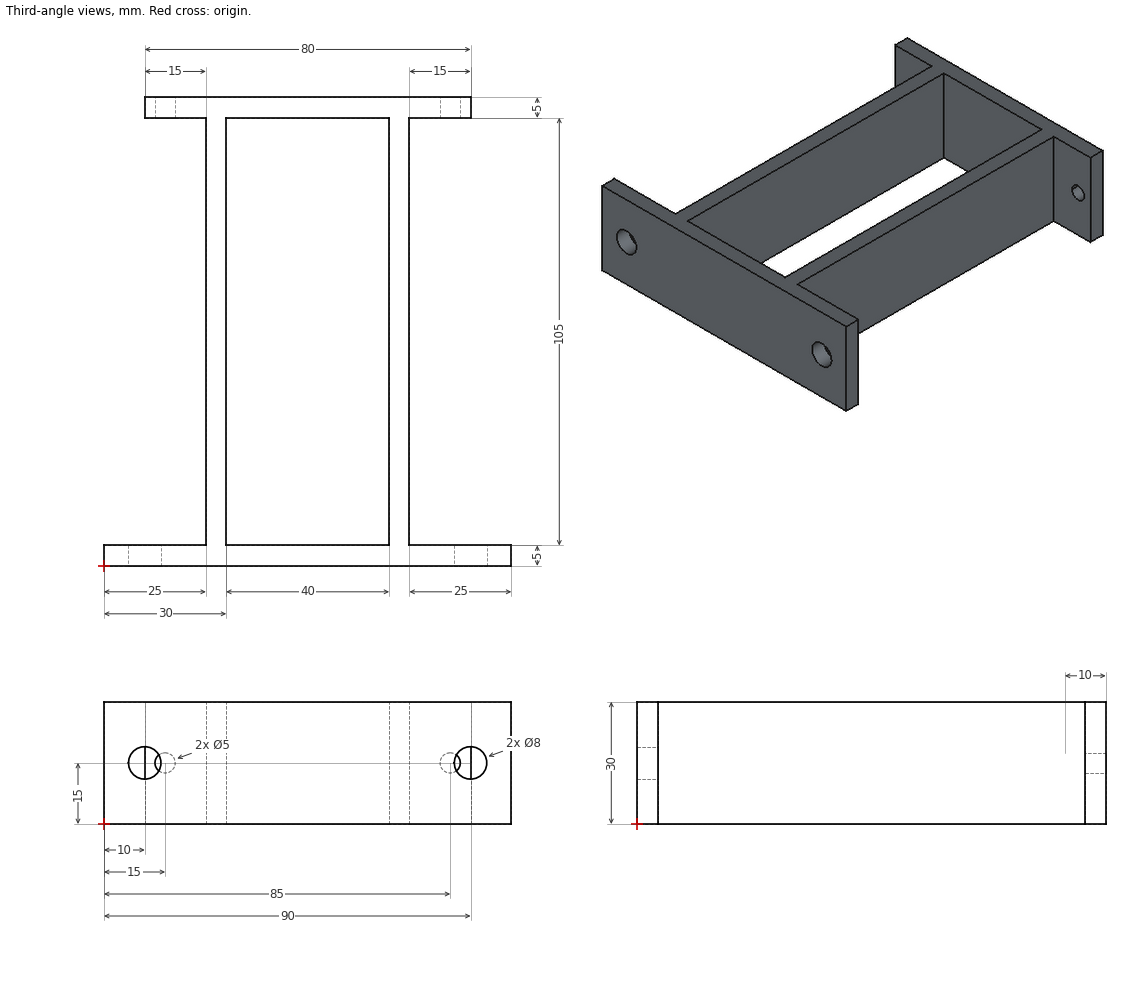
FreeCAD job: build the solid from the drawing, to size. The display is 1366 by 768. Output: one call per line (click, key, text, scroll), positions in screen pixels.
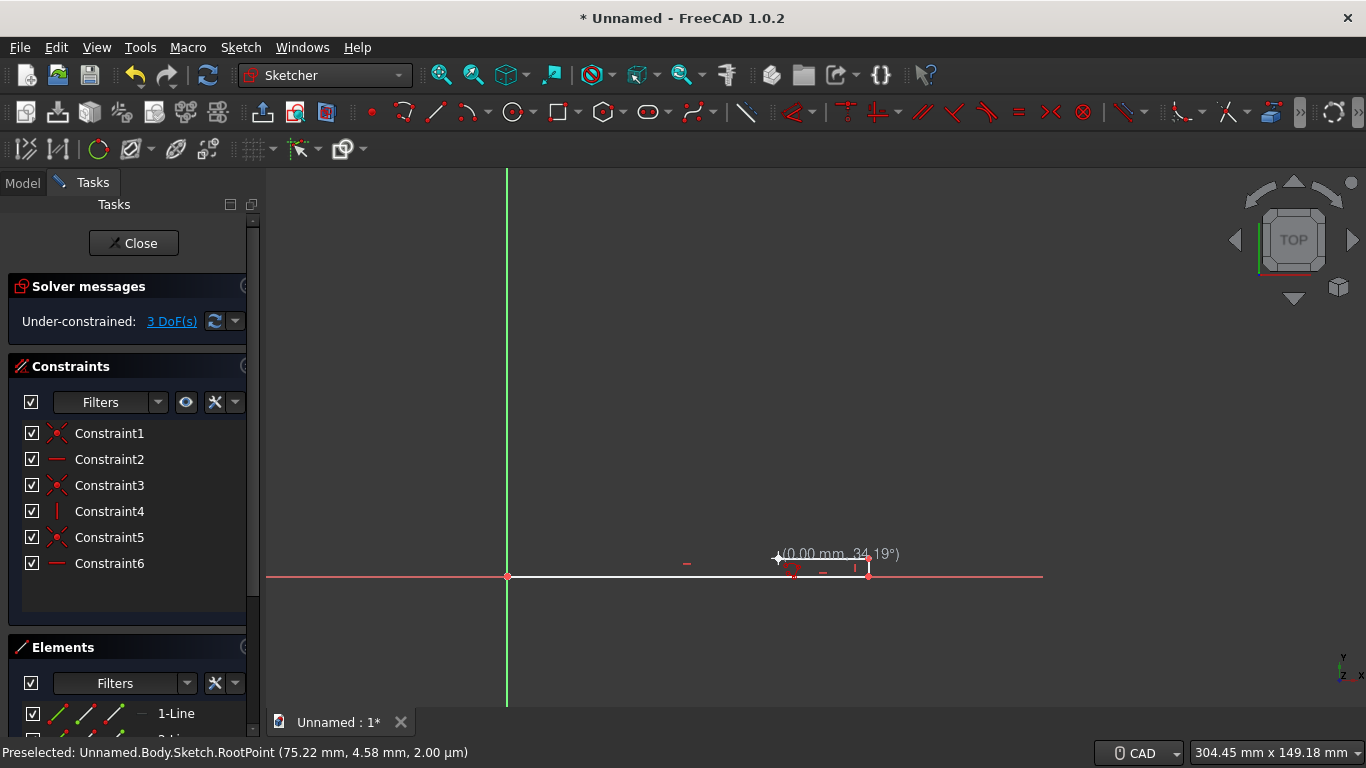
scroll(1017, 679, down, 1)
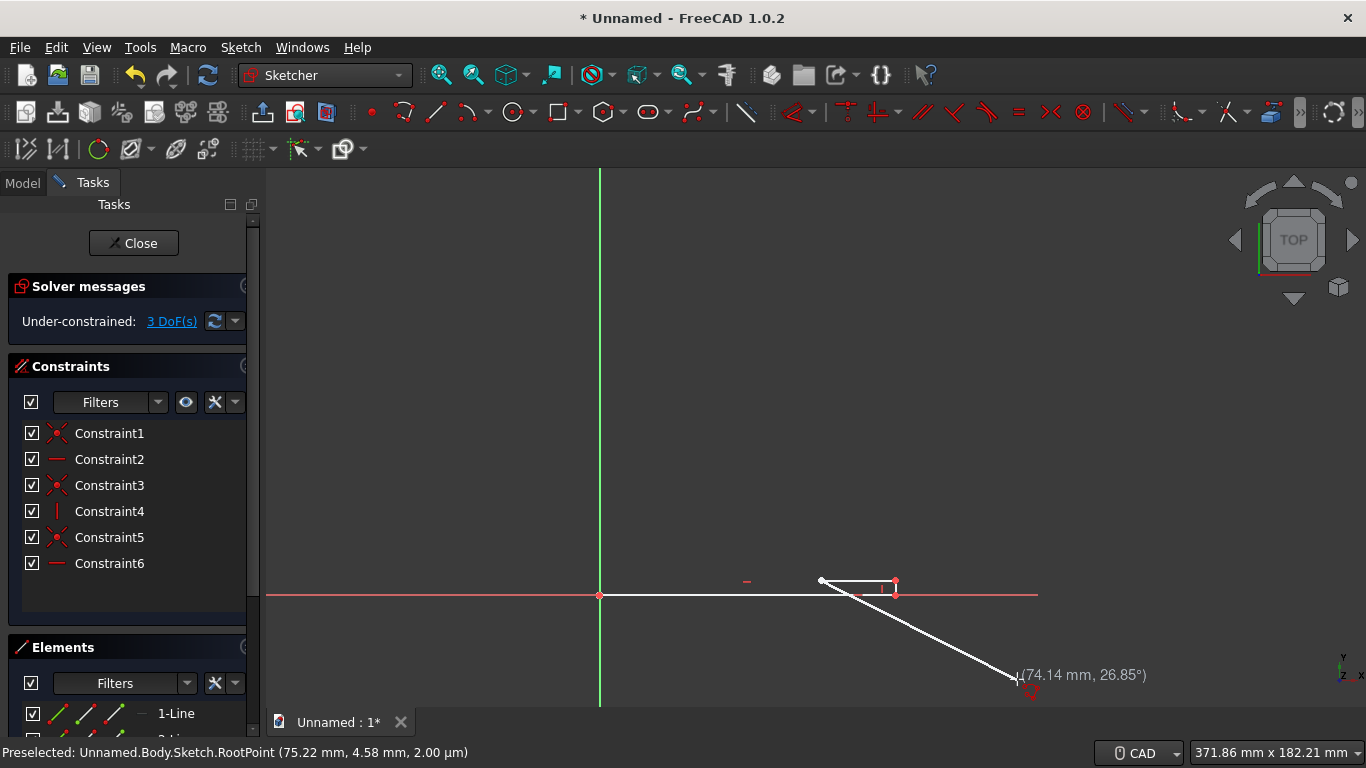
click(821, 270)
click(866, 270)
click(866, 255)
click(629, 255)
click(629, 270)
click(674, 270)
click(674, 581)
click(609, 581)
click(600, 595)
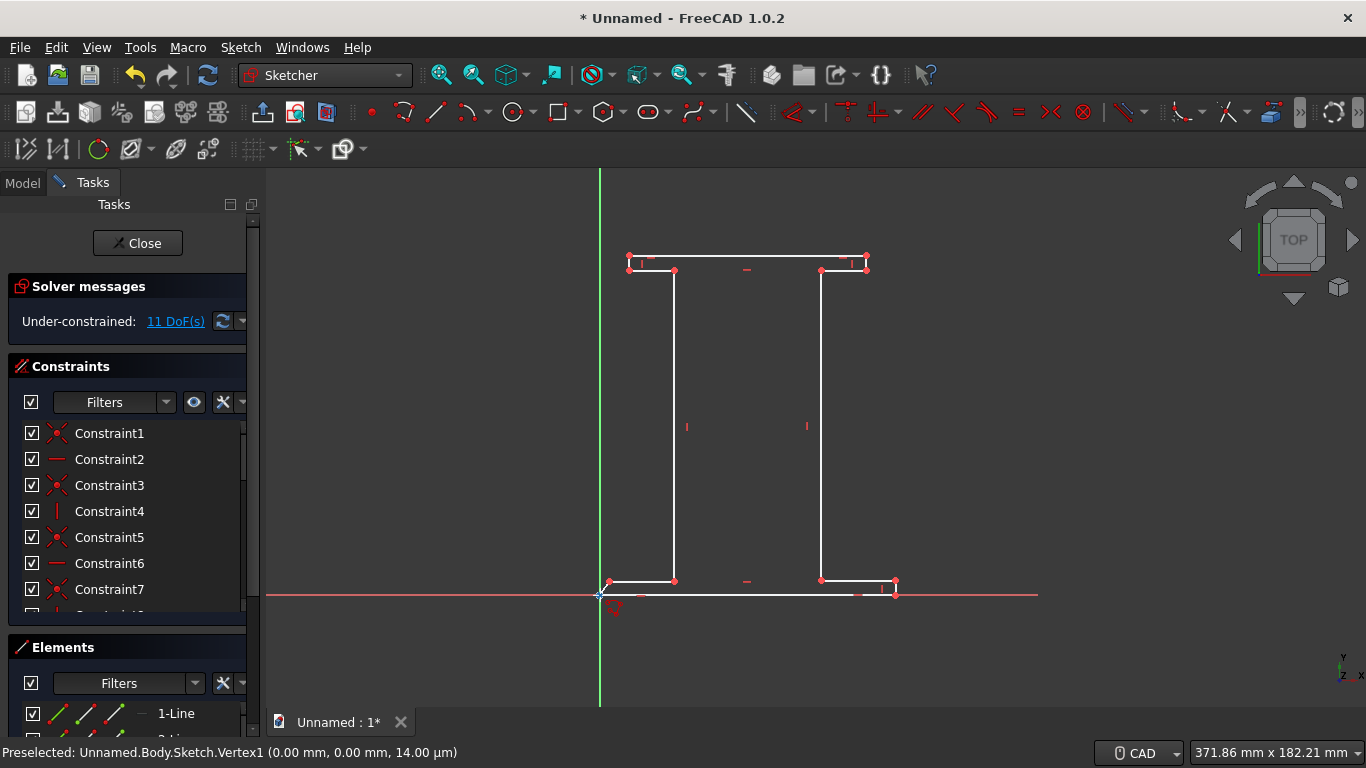
click(558, 112)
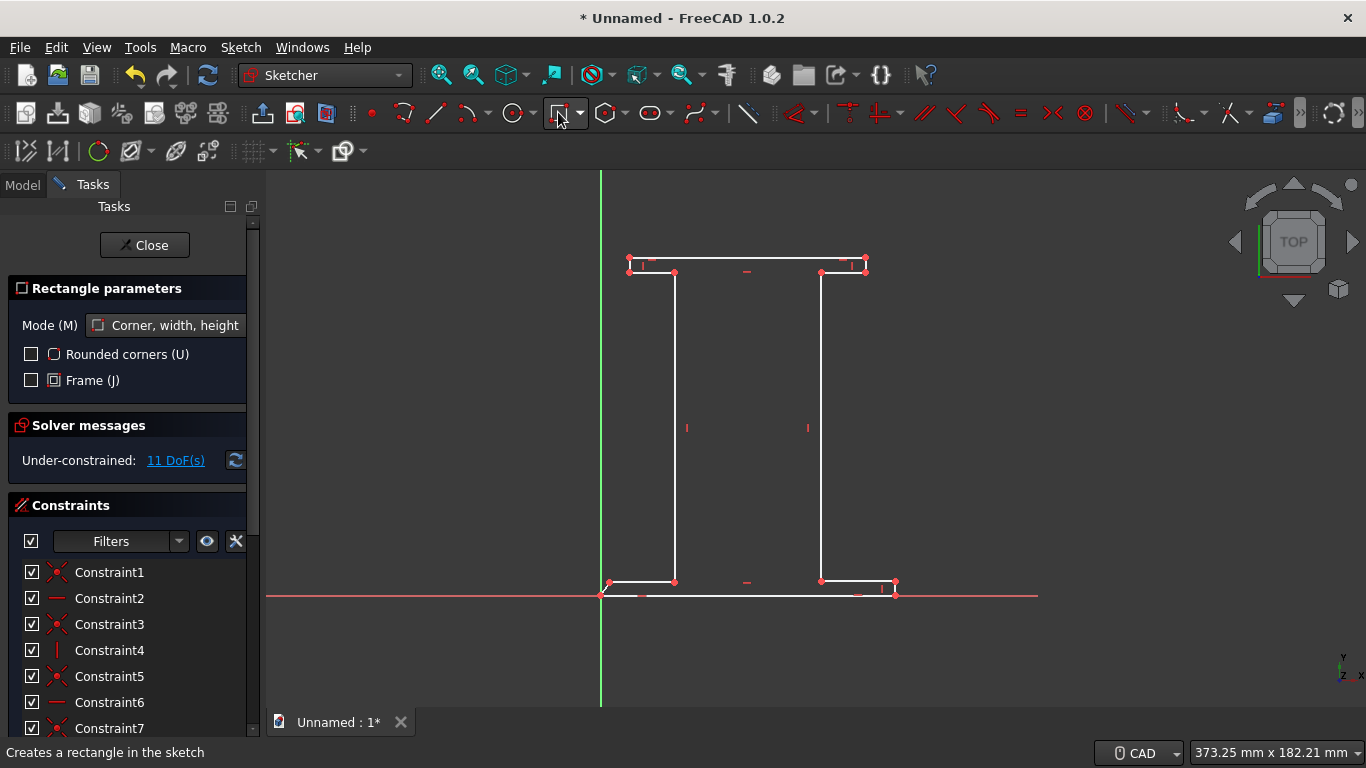
click(689, 272)
click(807, 581)
key(Escape)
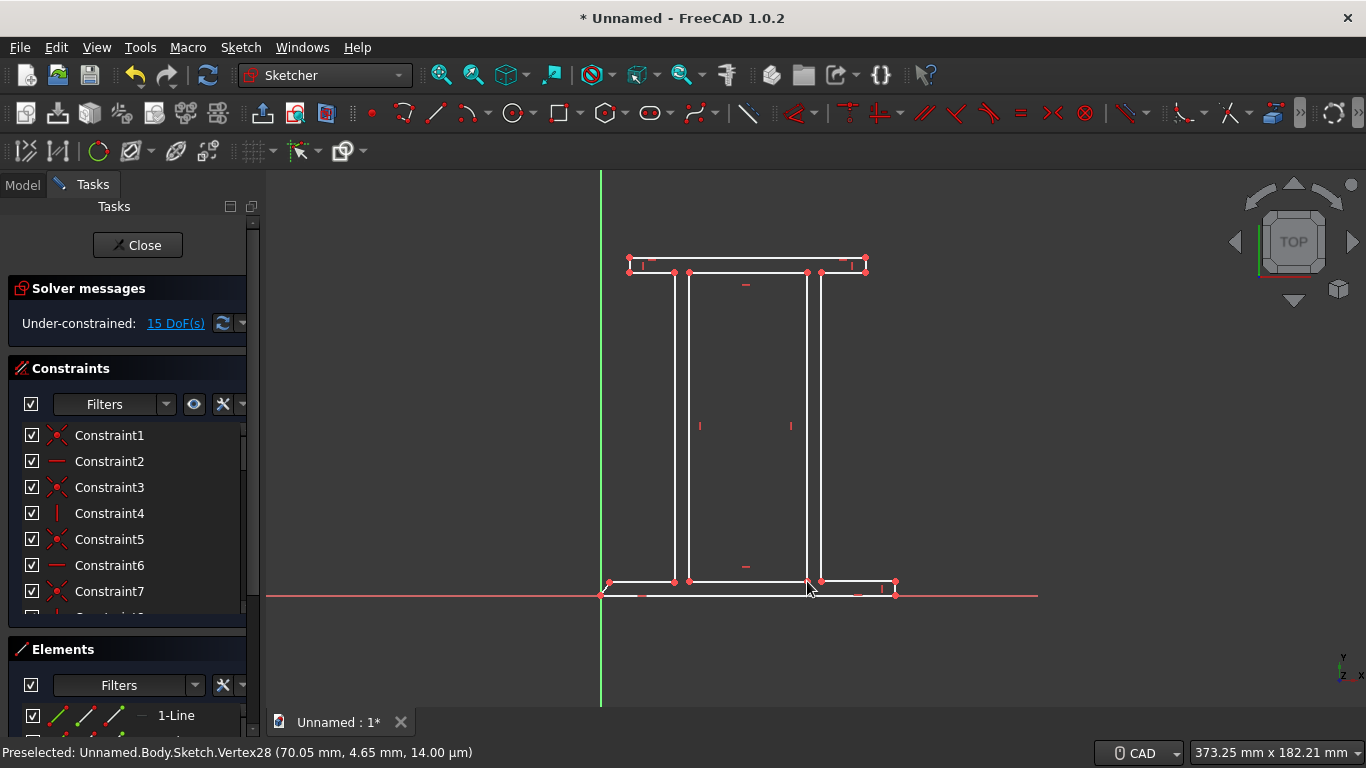
scroll(606, 588, up, 5)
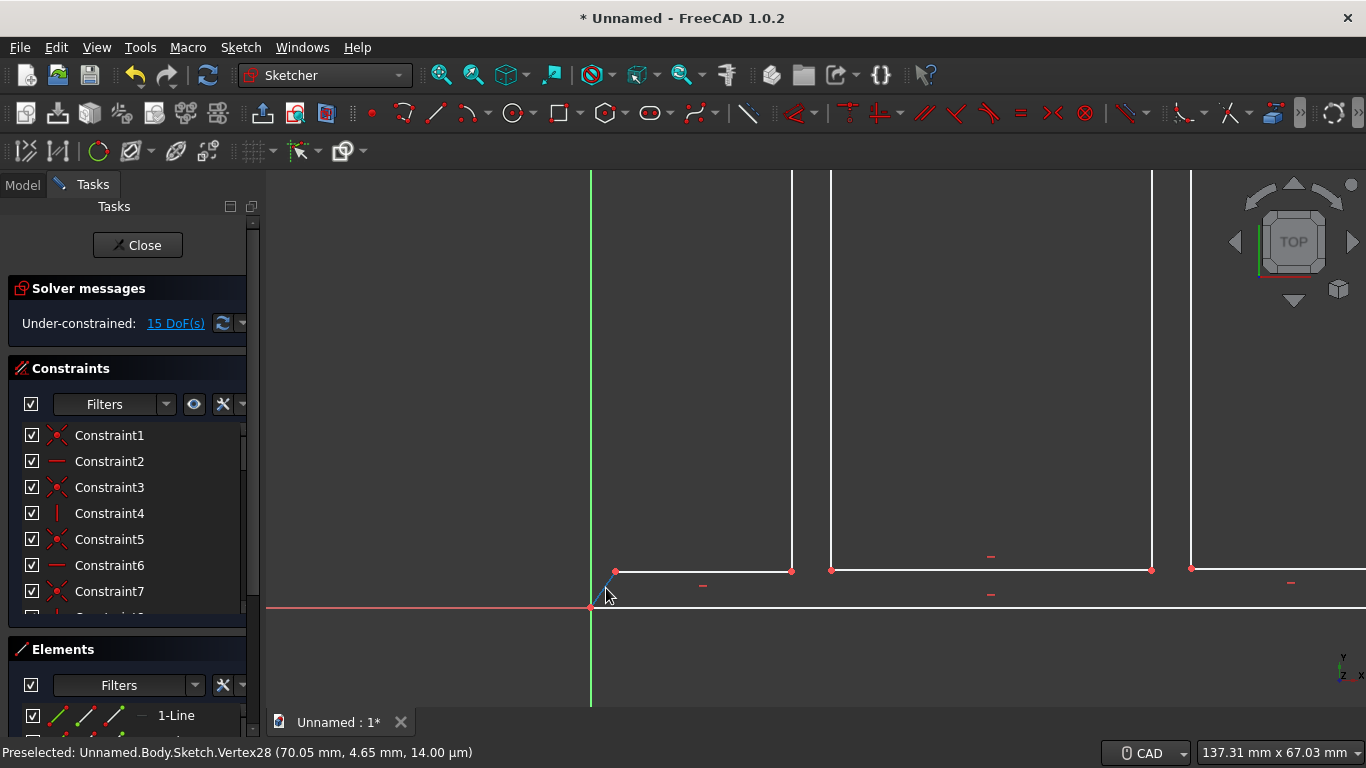
click(606, 586)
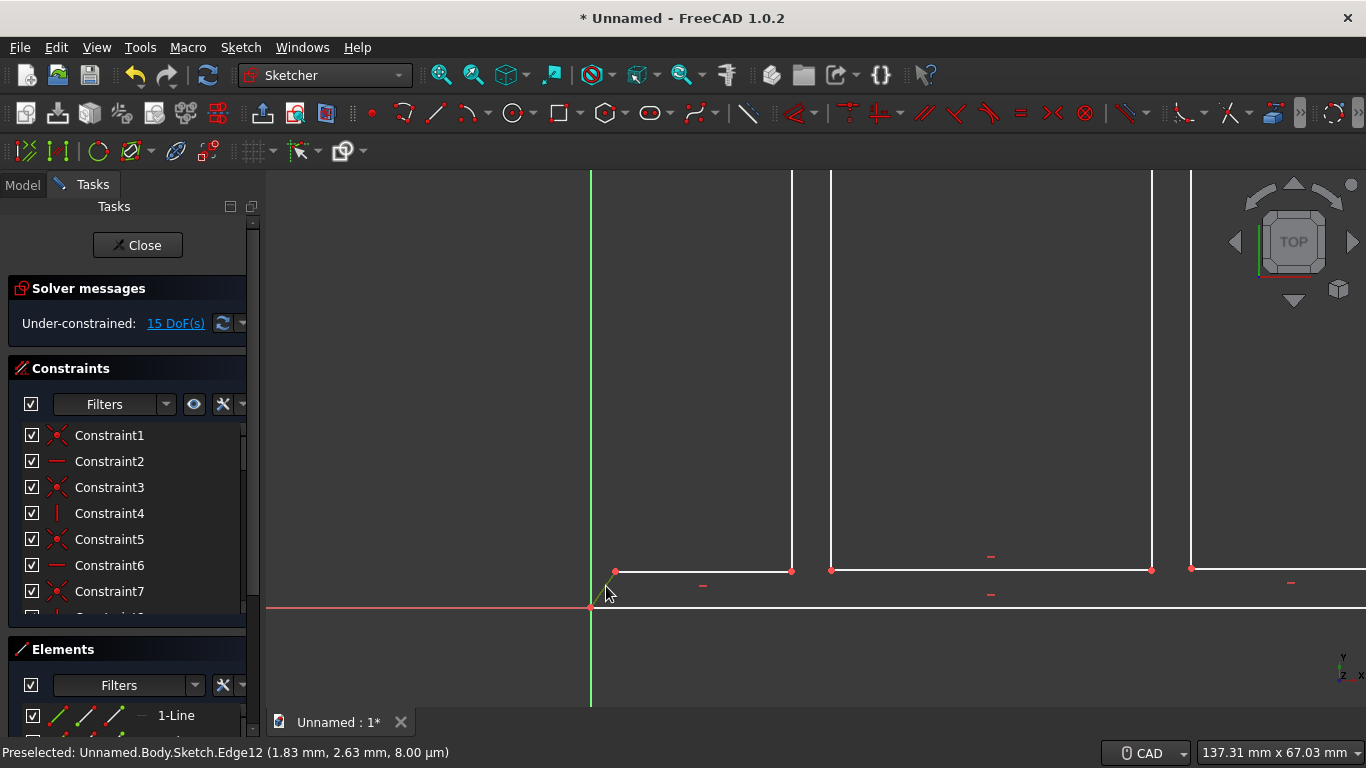
click(902, 114)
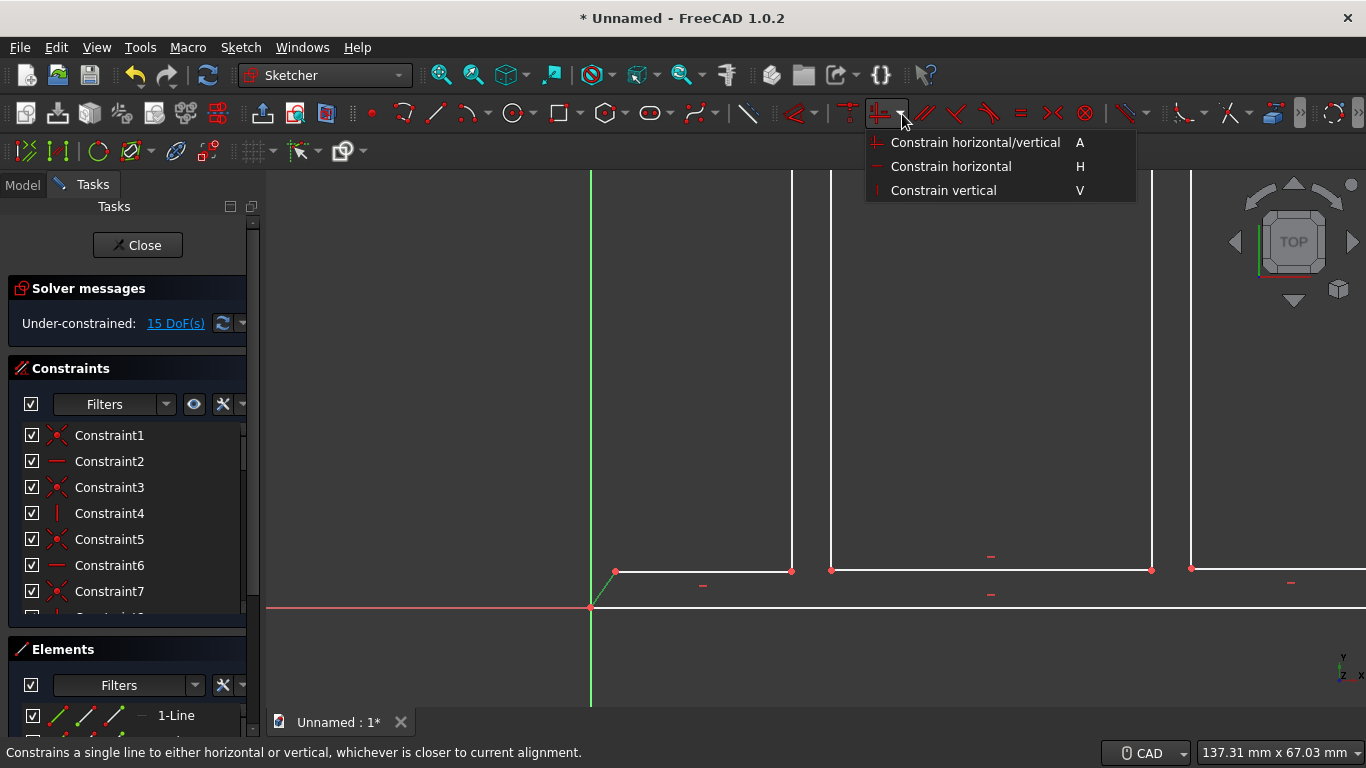
click(1001, 190)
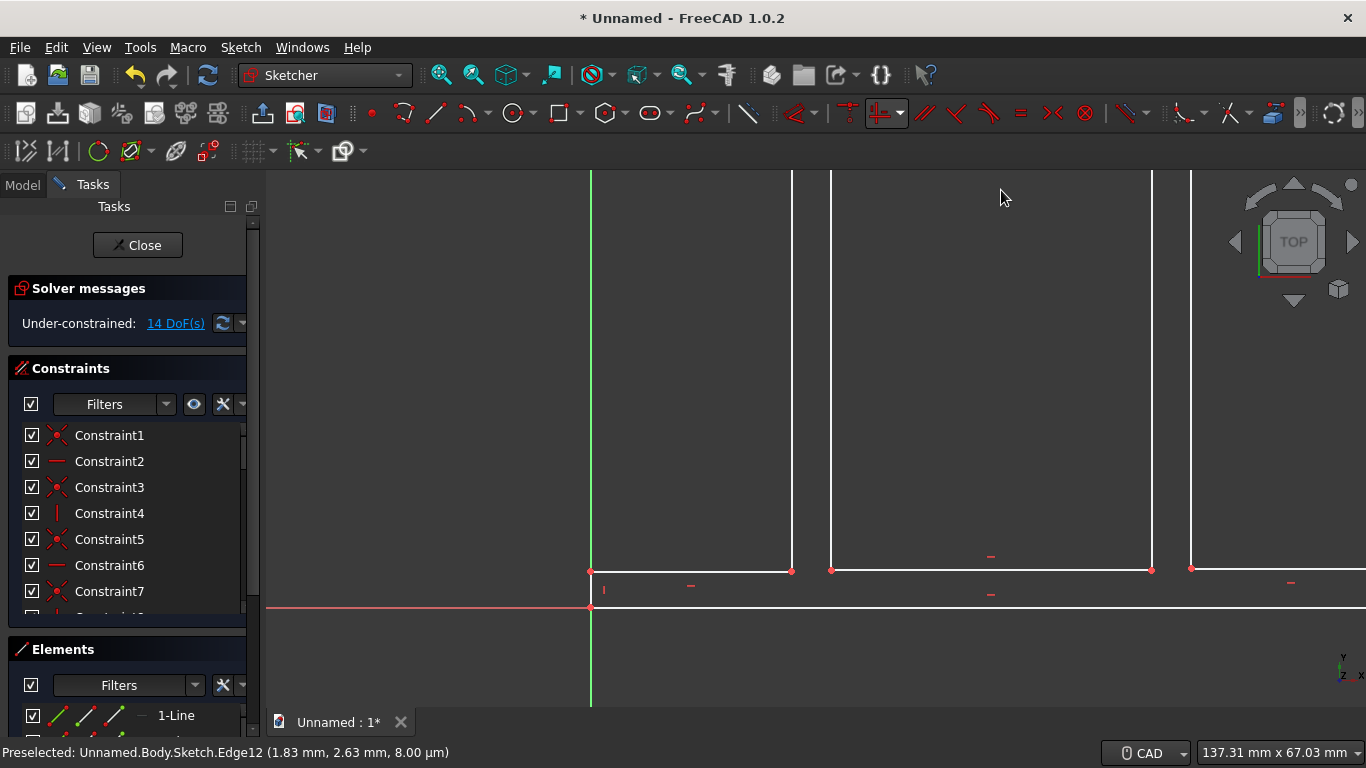
click(794, 114)